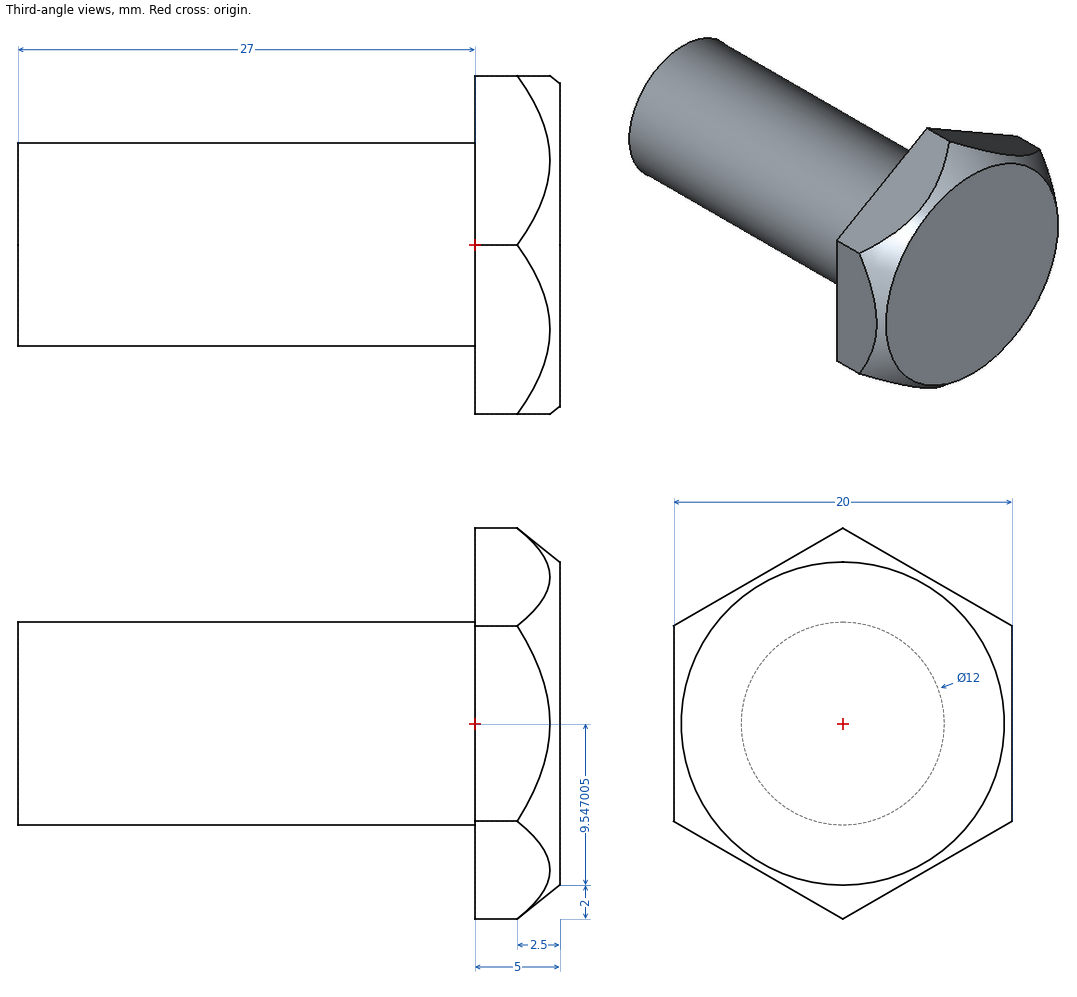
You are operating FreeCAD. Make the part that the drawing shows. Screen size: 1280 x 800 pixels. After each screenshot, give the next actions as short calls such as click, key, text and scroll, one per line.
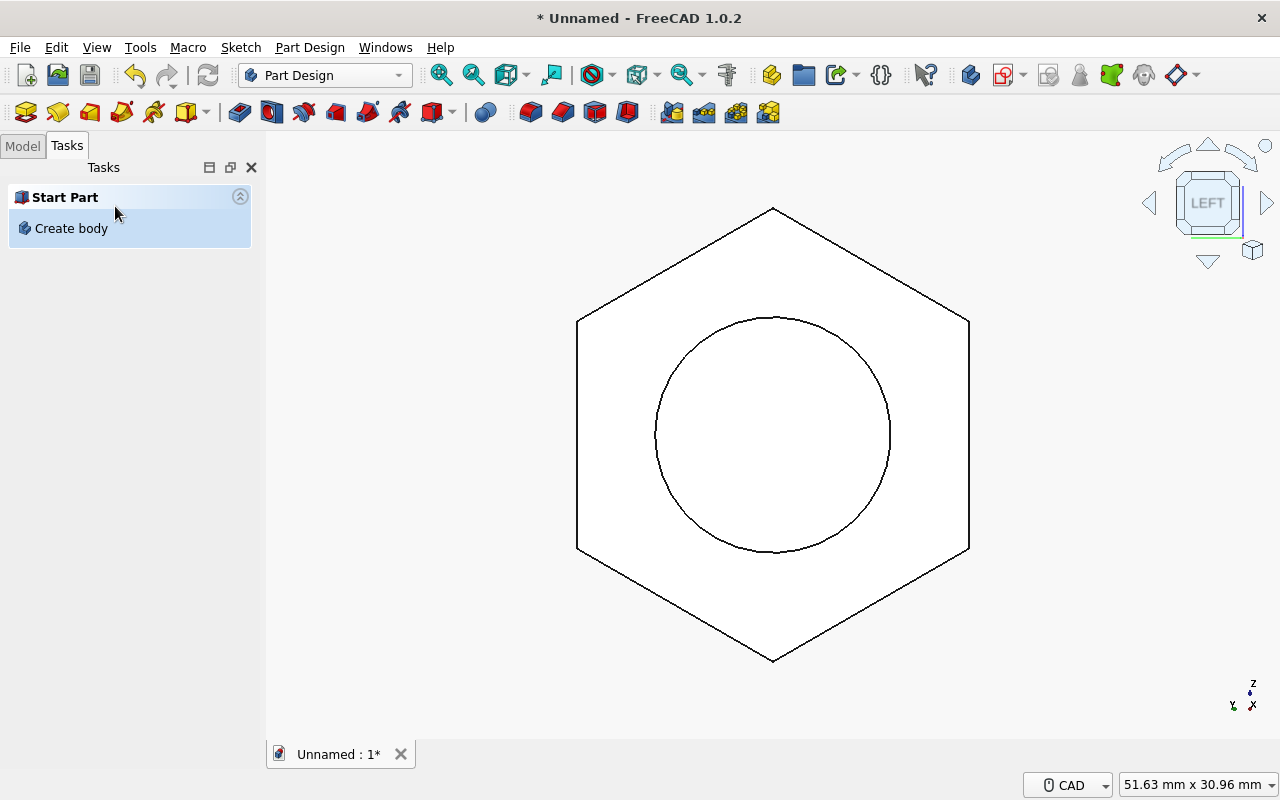
click(1004, 76)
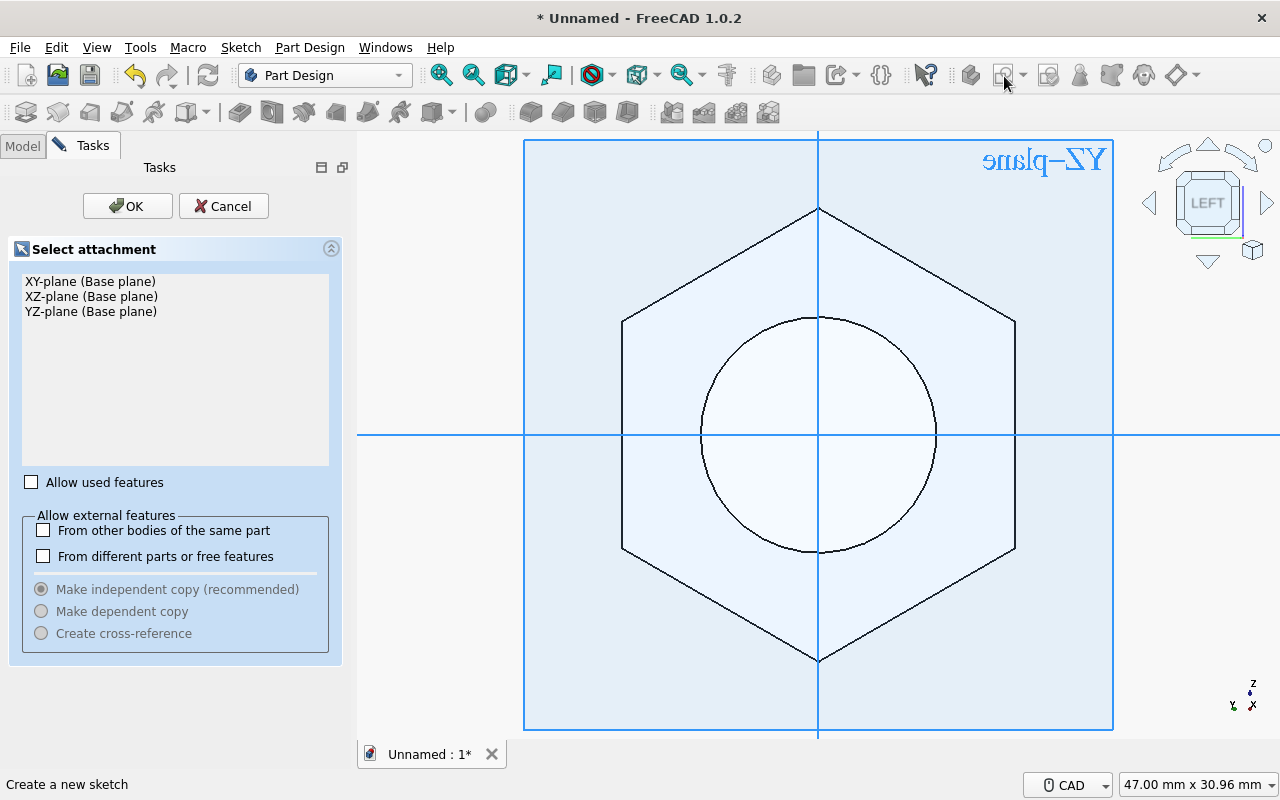
click(82, 296)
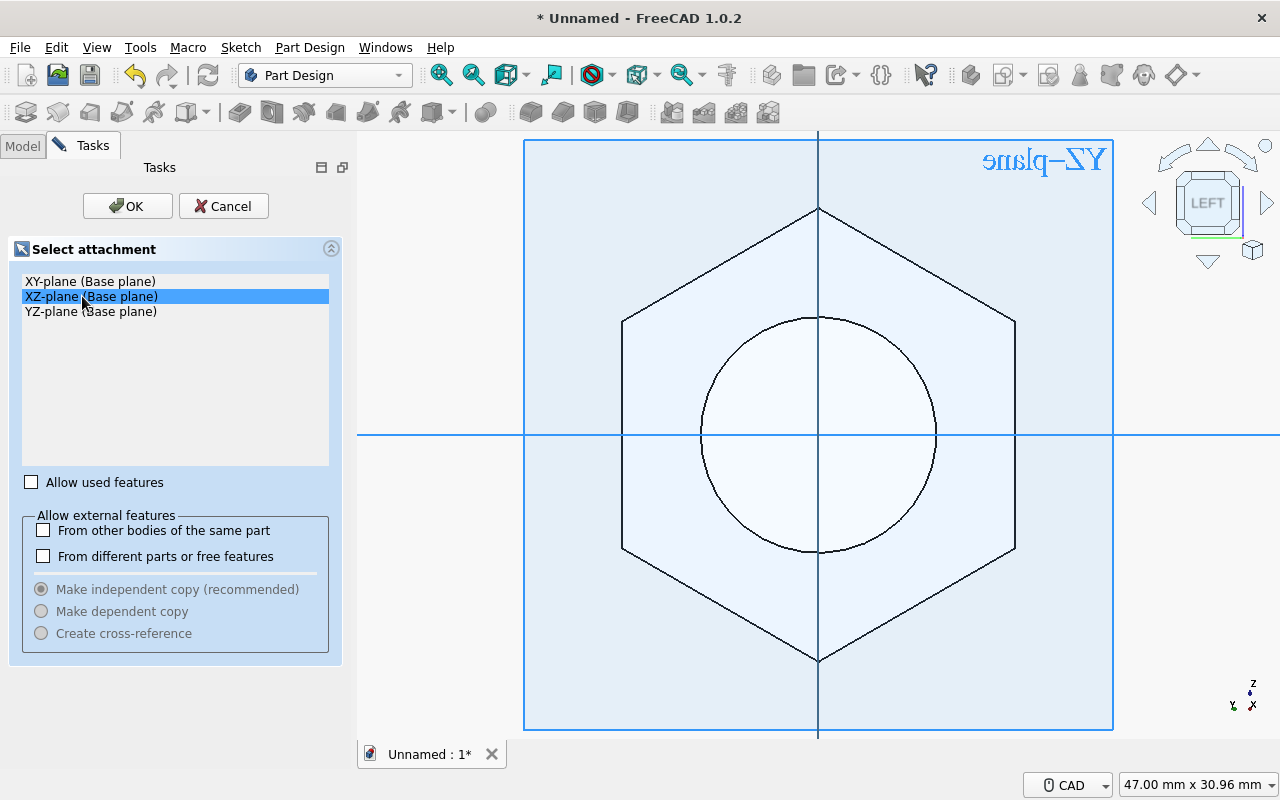
click(128, 206)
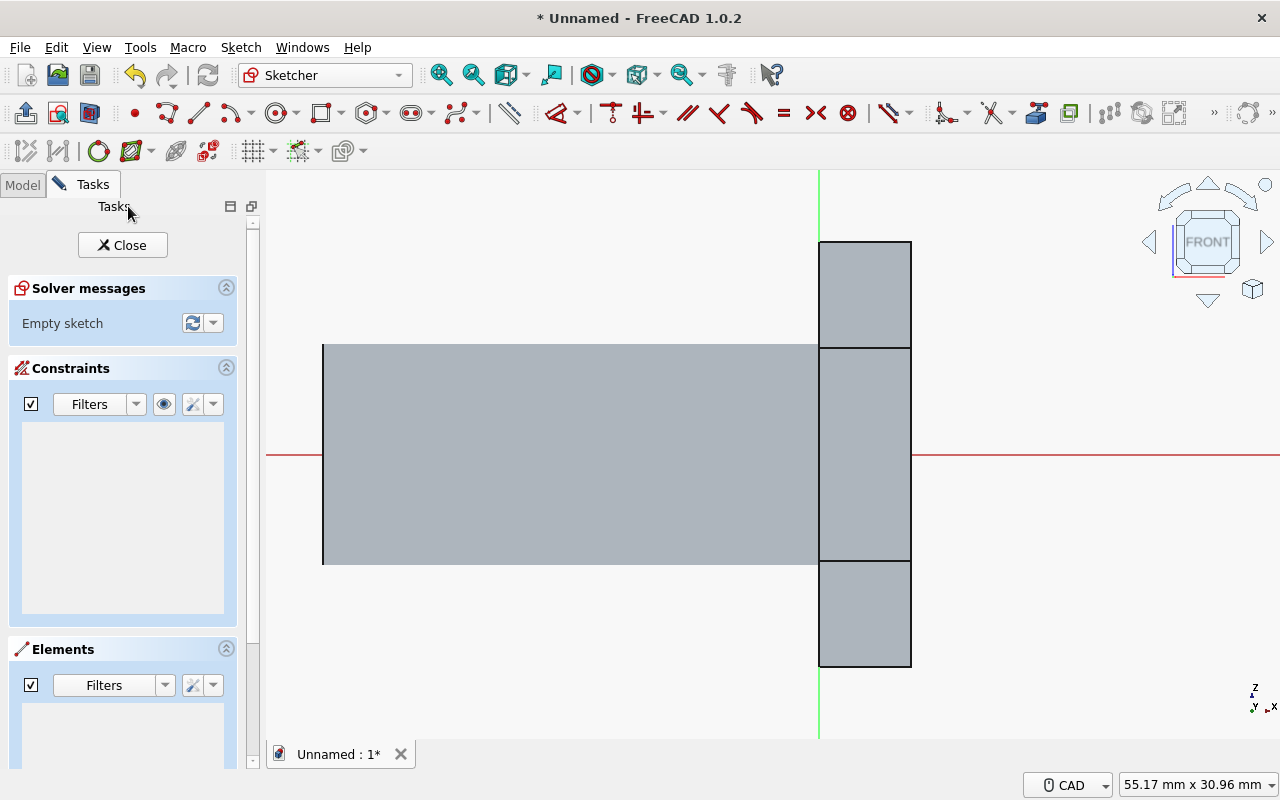
click(90, 114)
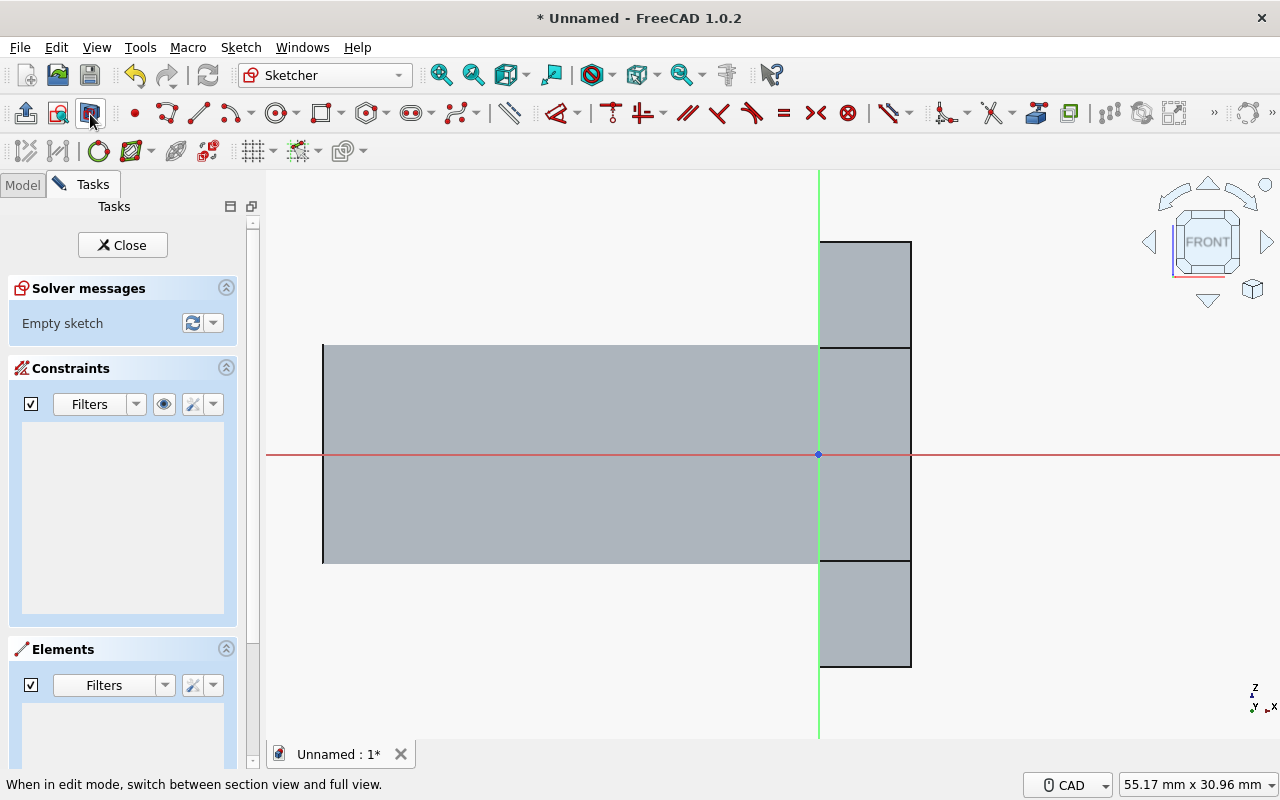
scroll(911, 673, up, 11)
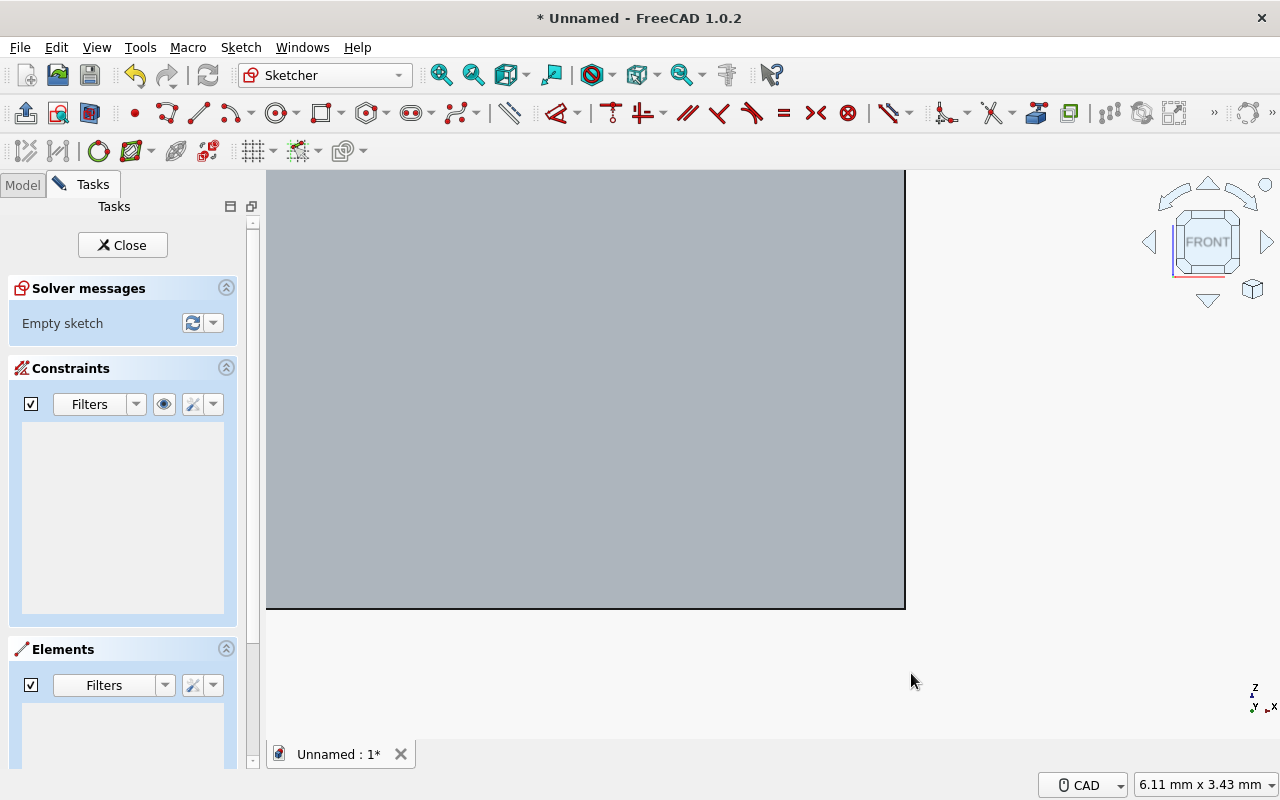
click(168, 114)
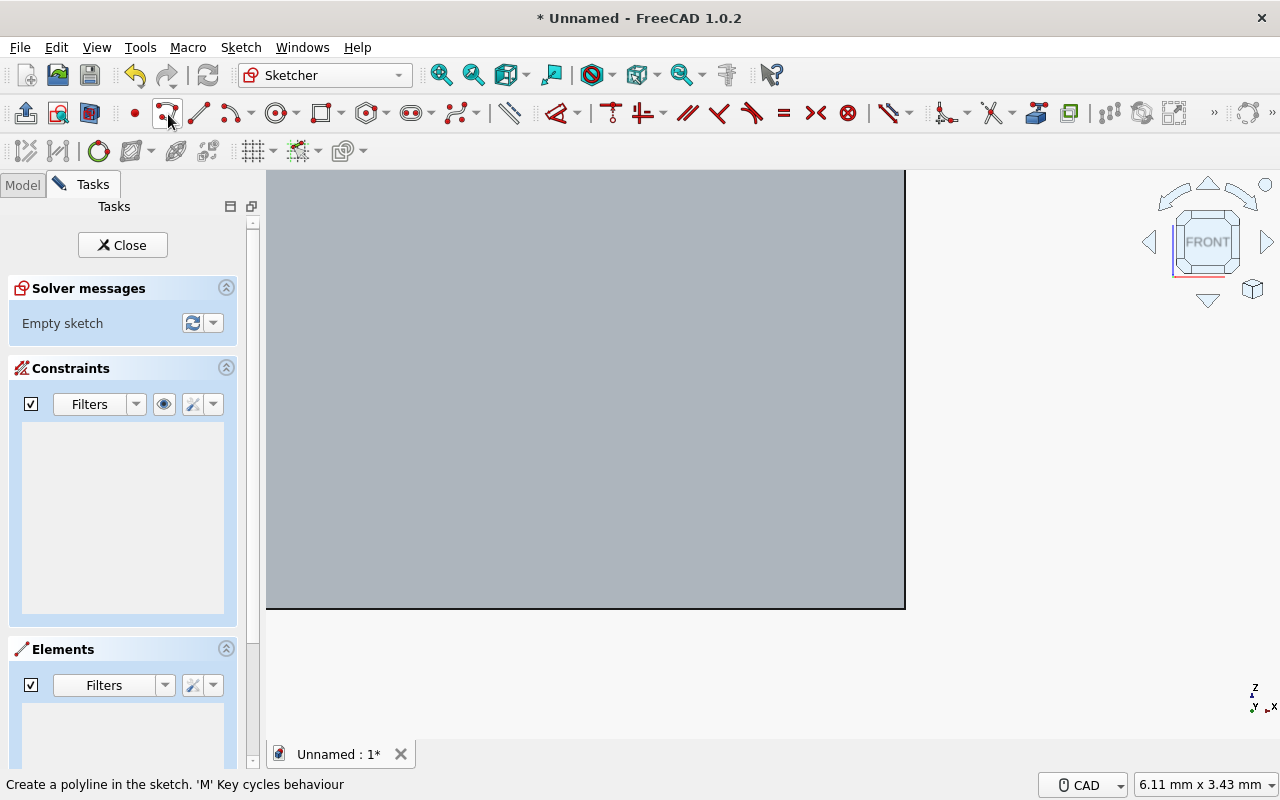
click(905, 278)
click(905, 609)
click(490, 609)
click(905, 279)
key(Escape)
key(Escape)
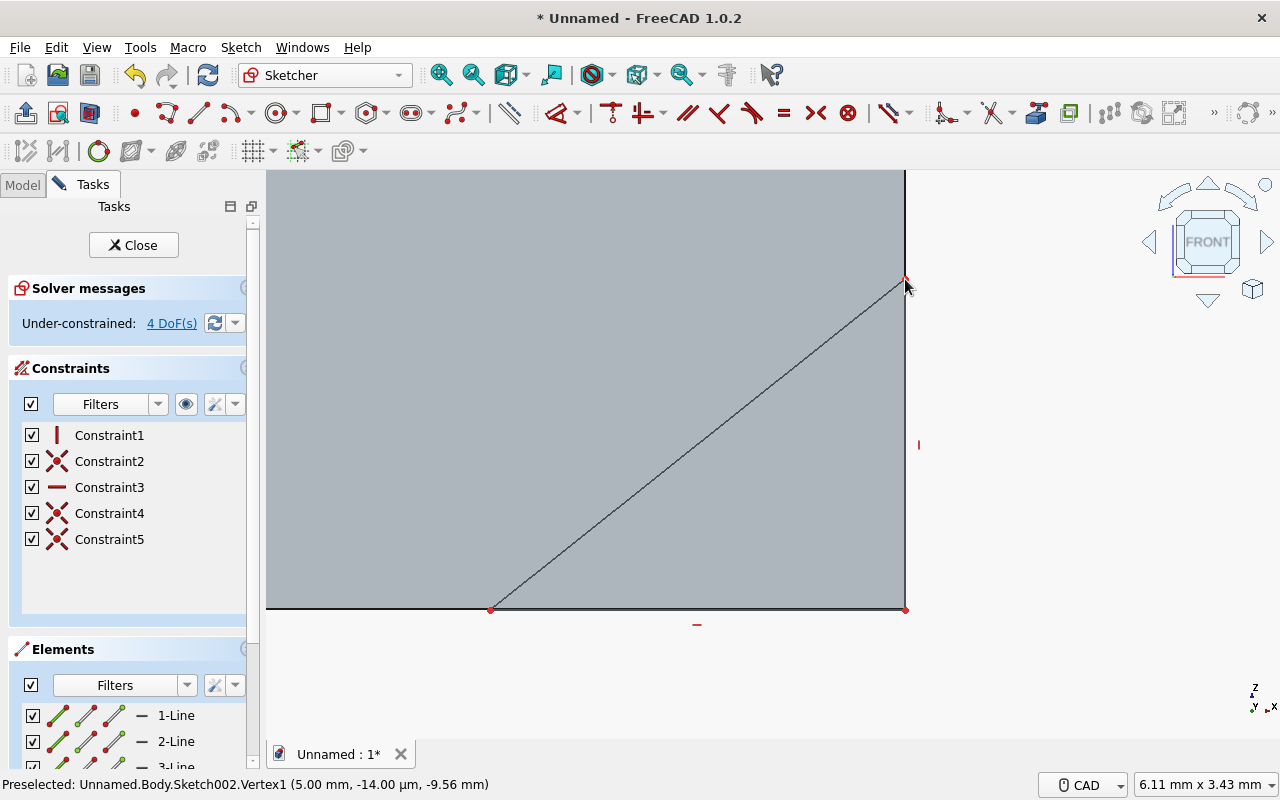
click(556, 114)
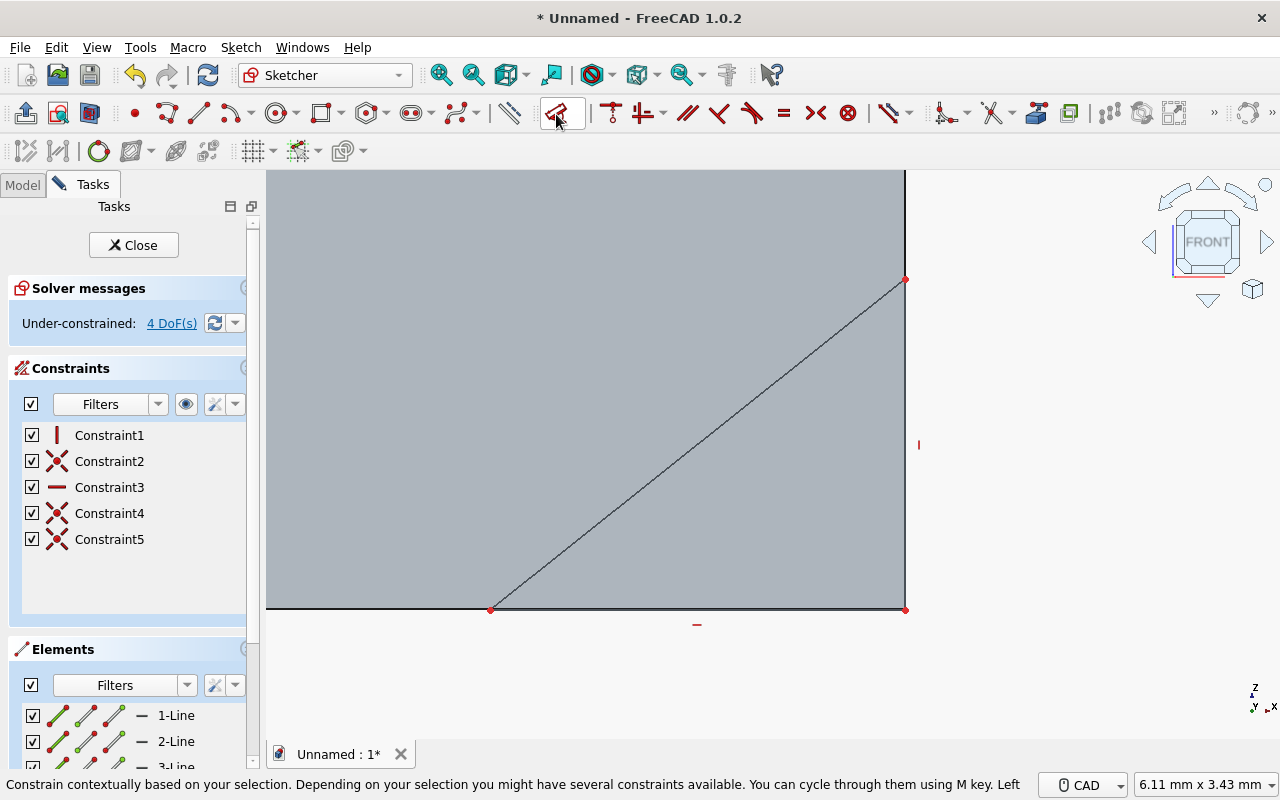
click(905, 378)
click(939, 445)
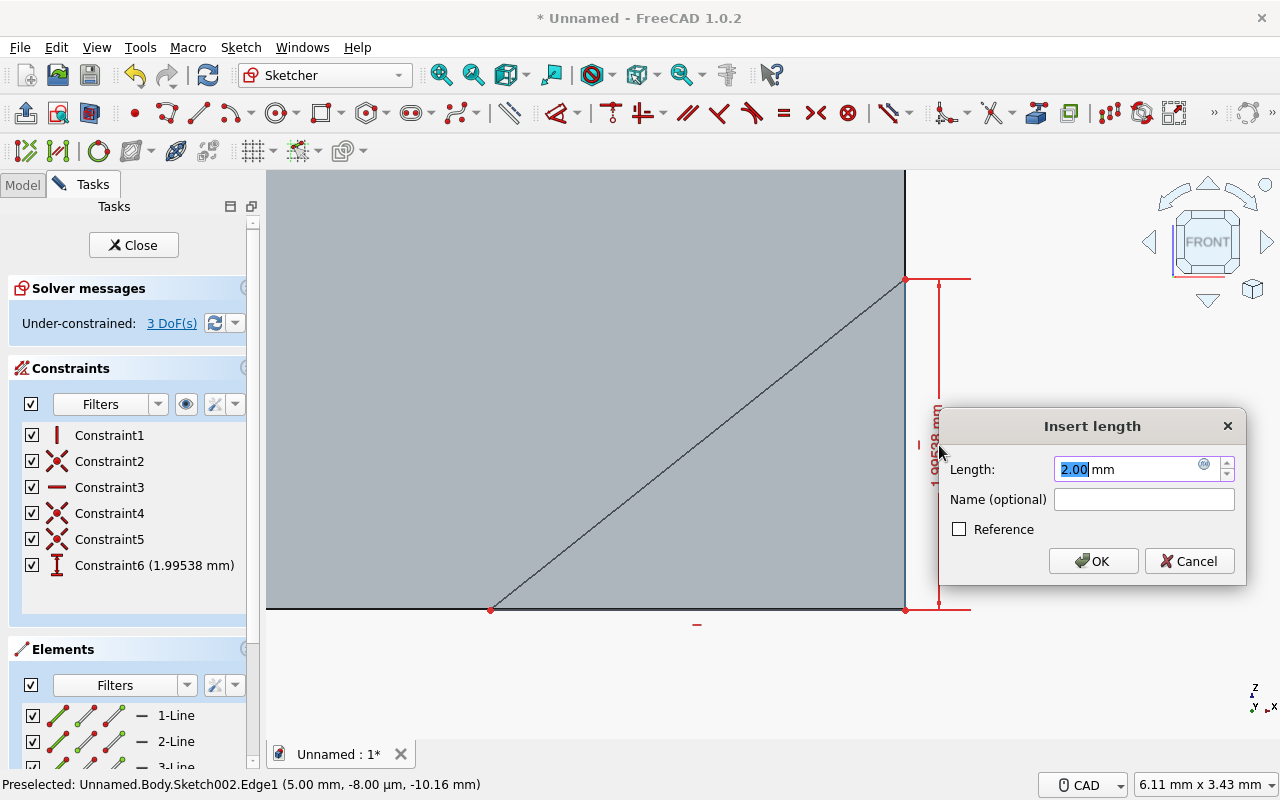
text(2)
key(Return)